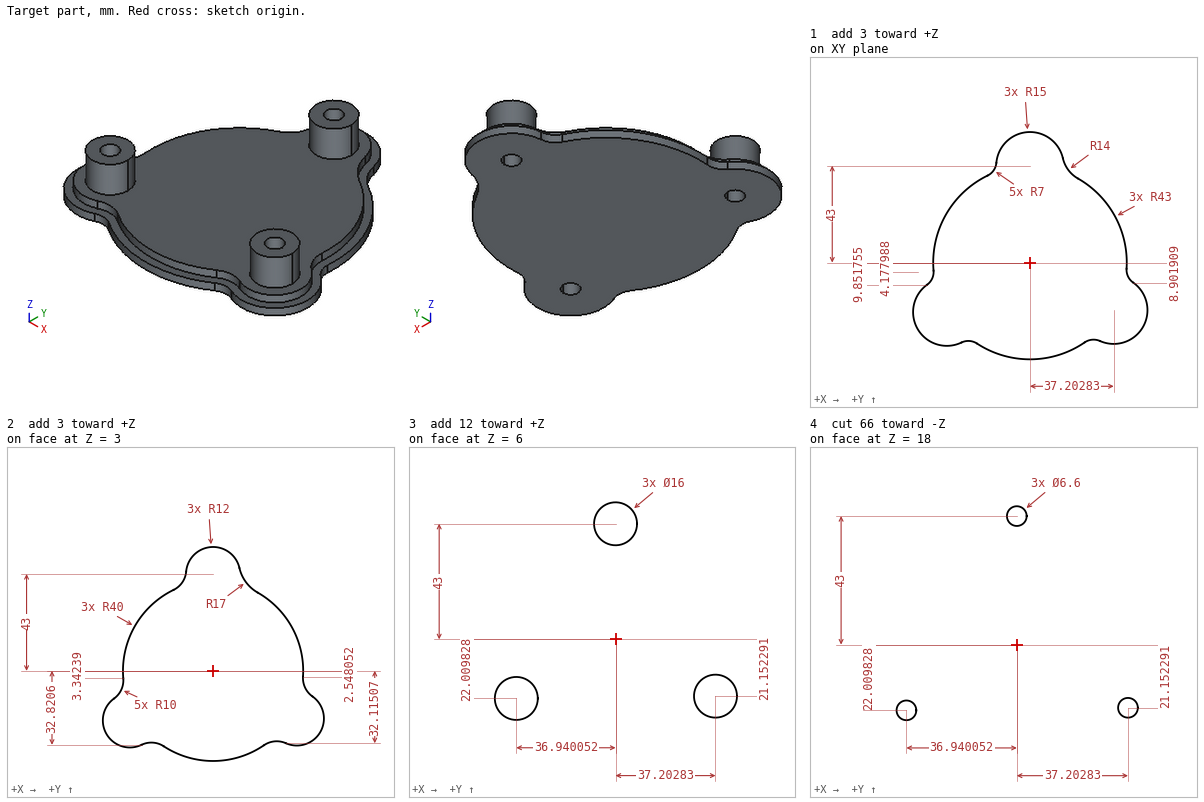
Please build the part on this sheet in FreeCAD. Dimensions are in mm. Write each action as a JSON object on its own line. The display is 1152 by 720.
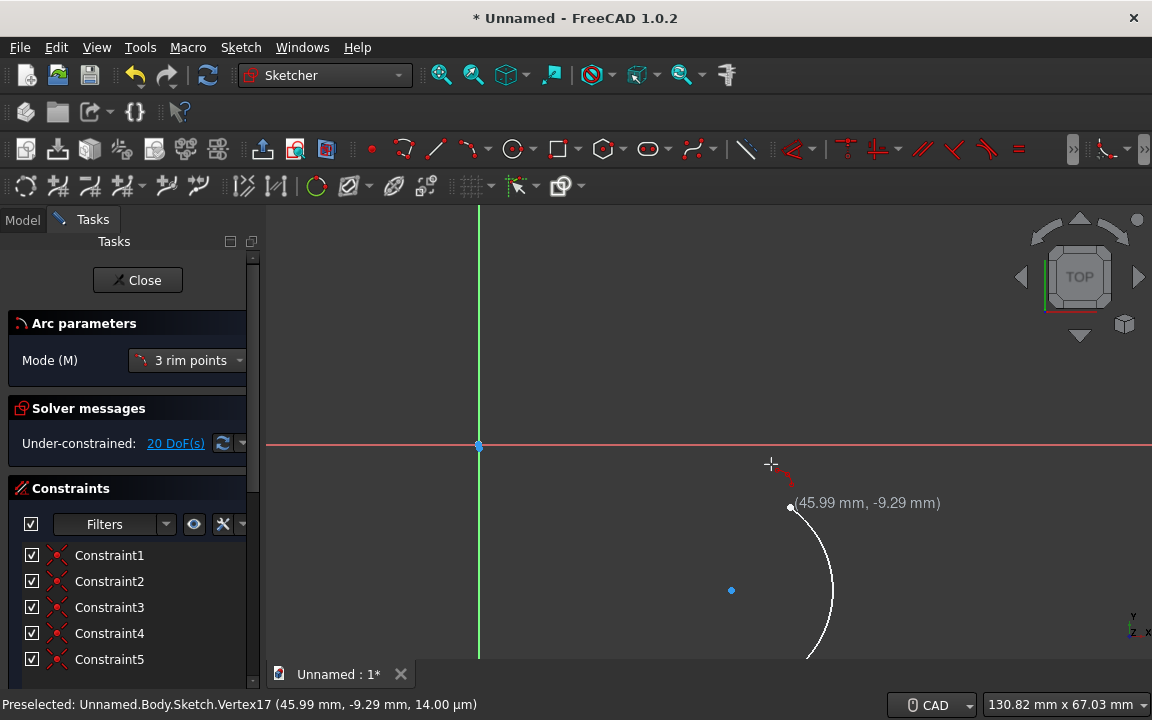
{"action": "left_click", "coordinate": [769, 463]}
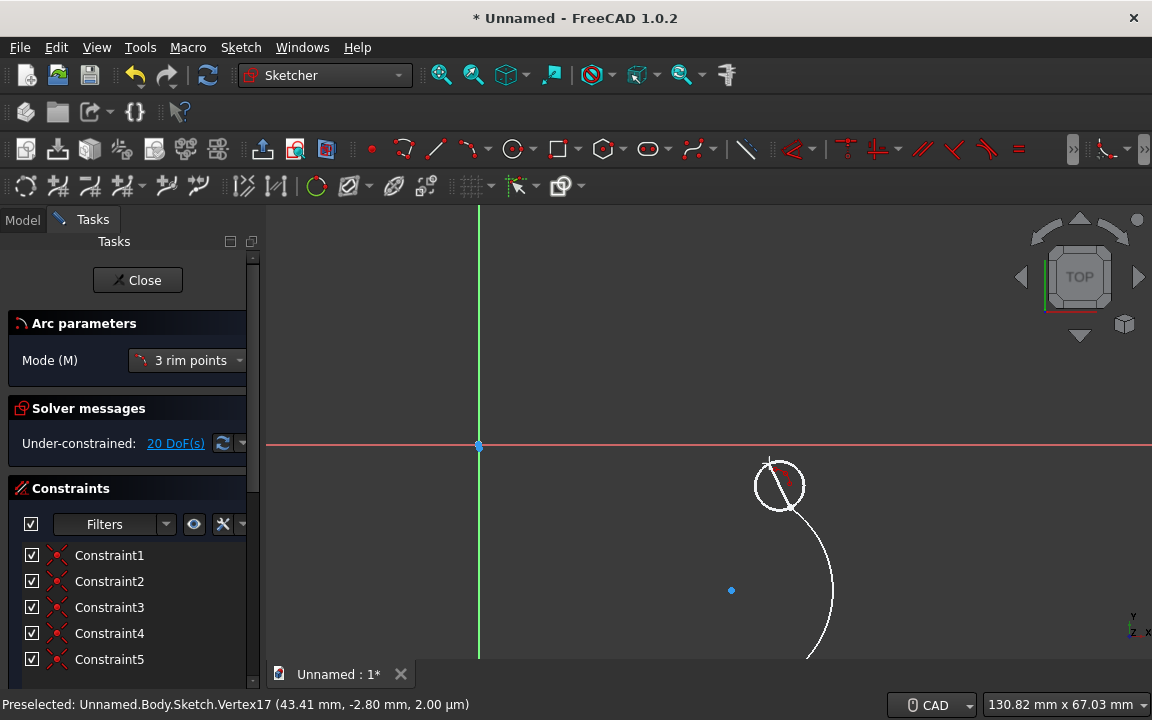
{"action": "scroll", "coordinate": [774, 487], "scroll_direction": "up", "scroll_amount": 5}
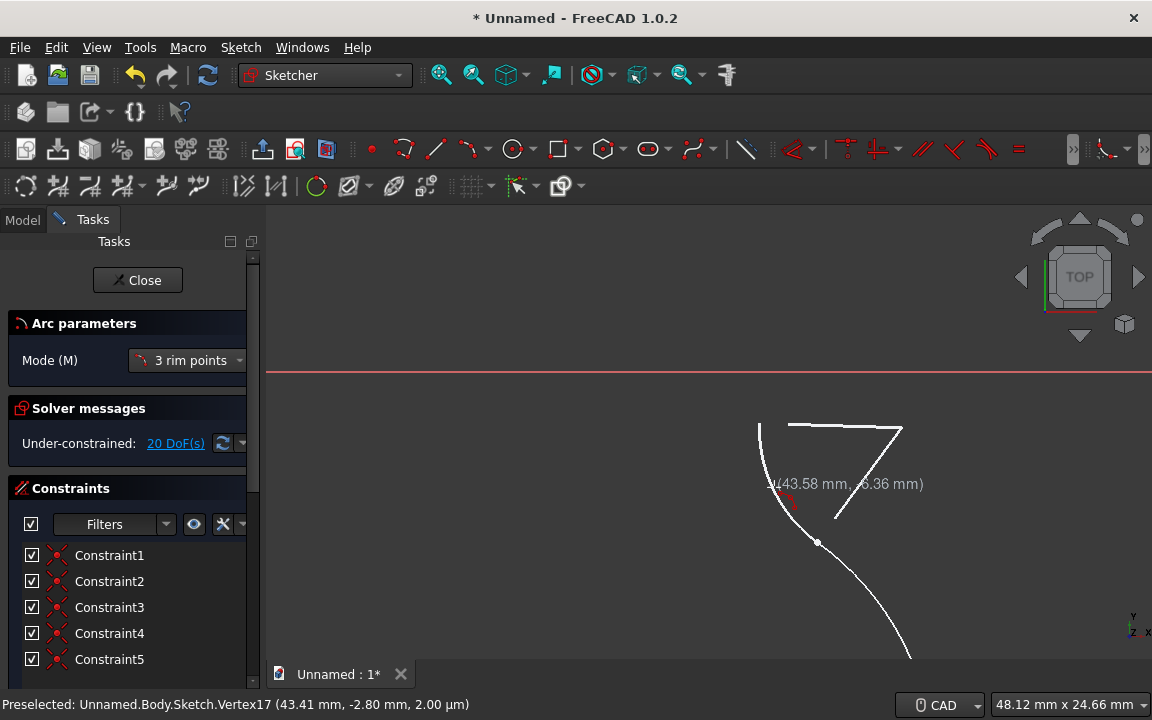
{"action": "left_click", "coordinate": [773, 486]}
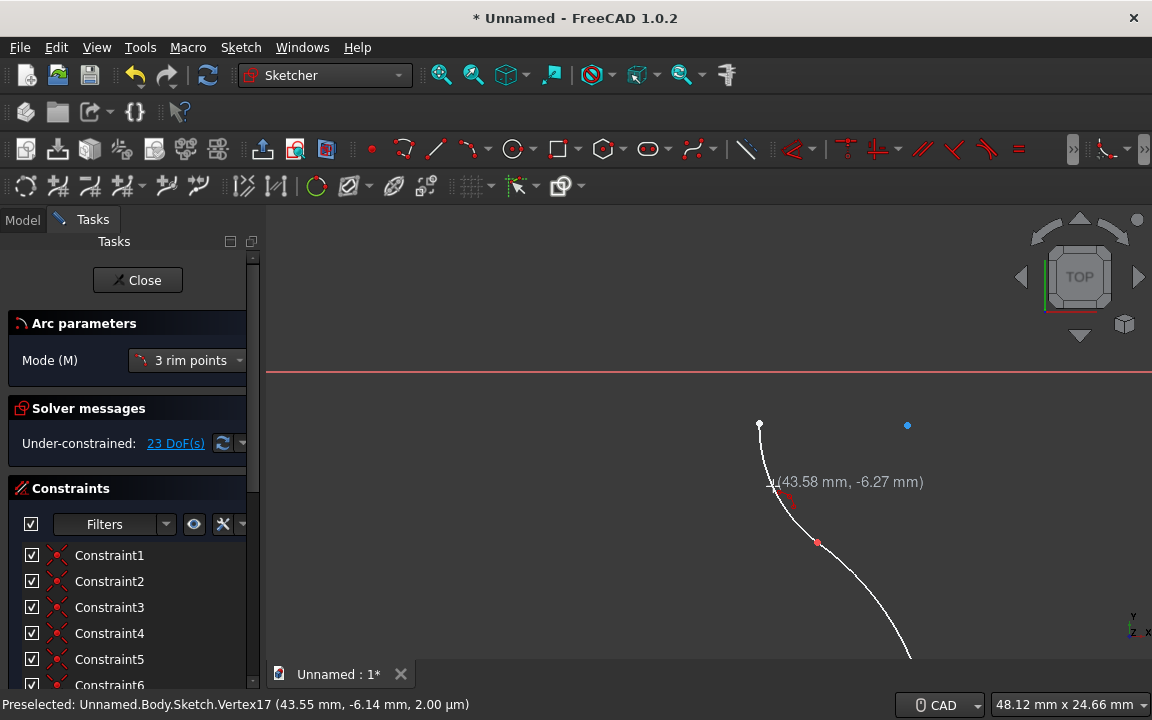
{"action": "scroll", "coordinate": [772, 471], "scroll_direction": "down", "scroll_amount": 9}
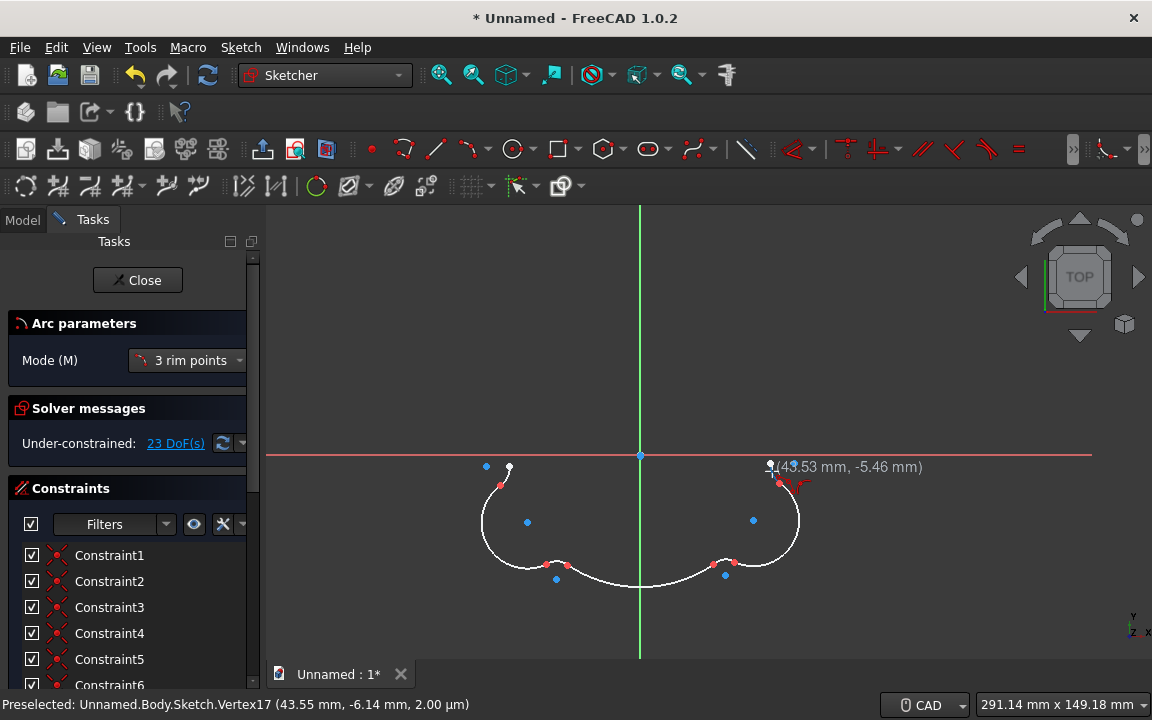
{"action": "scroll", "coordinate": [771, 463], "scroll_direction": "up", "scroll_amount": 4}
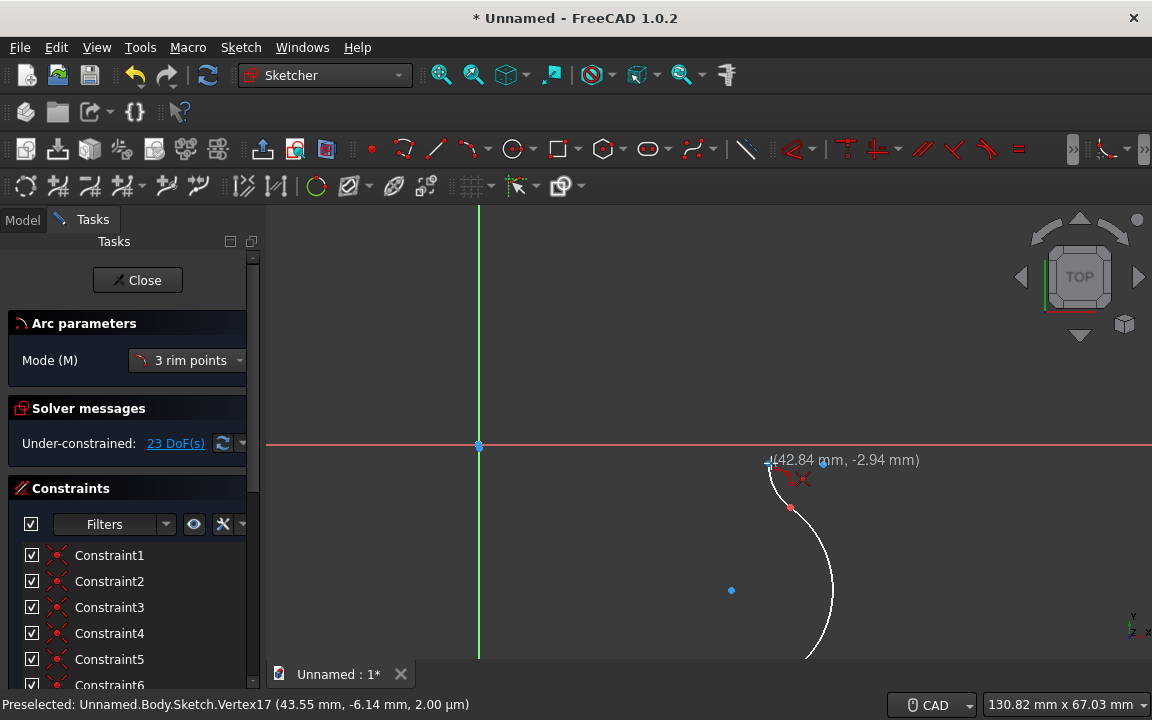
{"action": "left_click", "coordinate": [769, 464]}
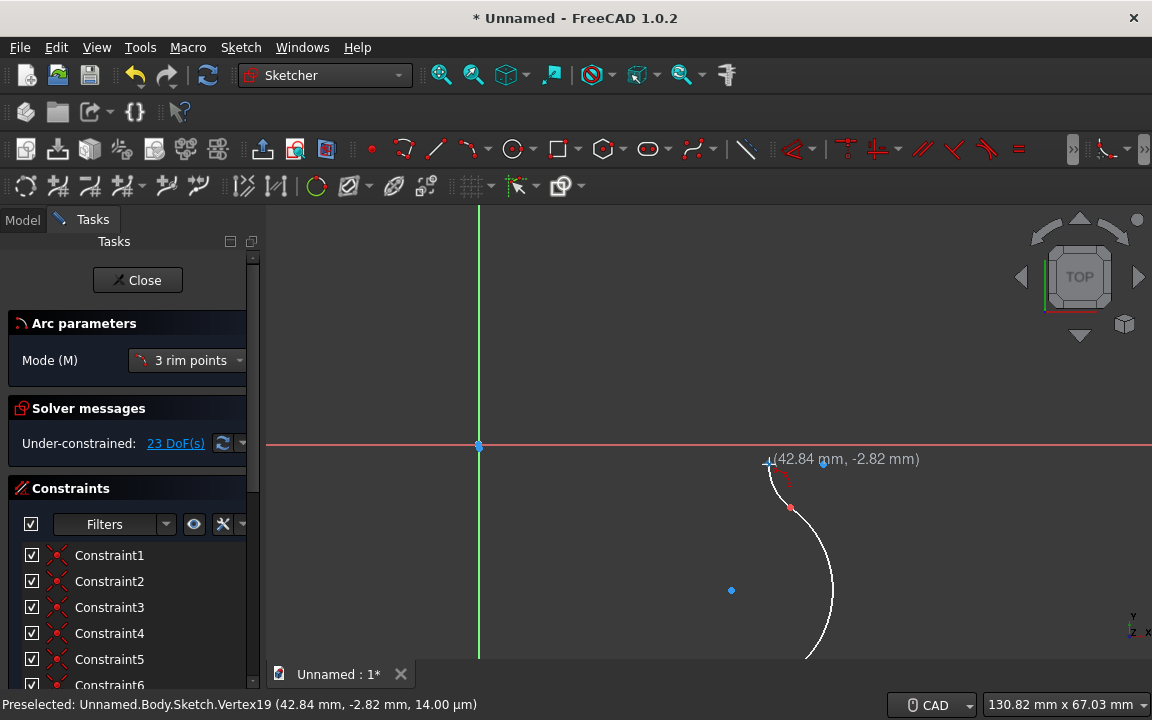
{"action": "scroll", "coordinate": [771, 463], "scroll_direction": "down", "scroll_amount": 4}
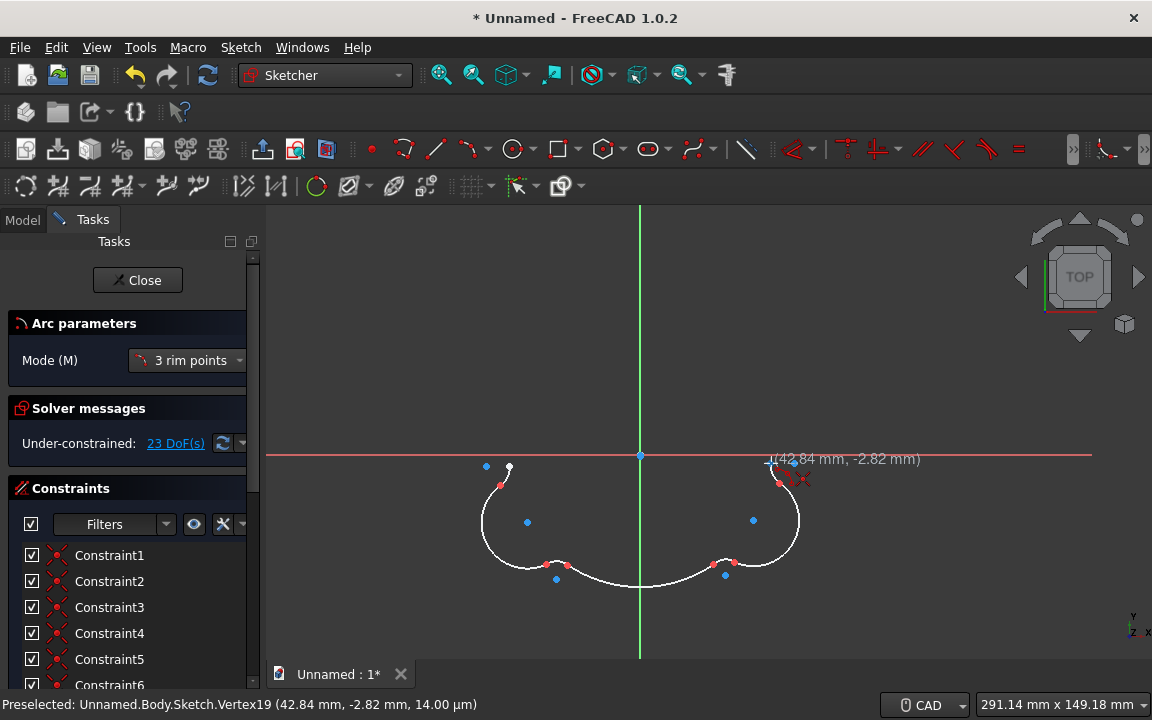
{"action": "left_click", "coordinate": [705, 341]}
{"action": "left_click", "coordinate": [755, 393]}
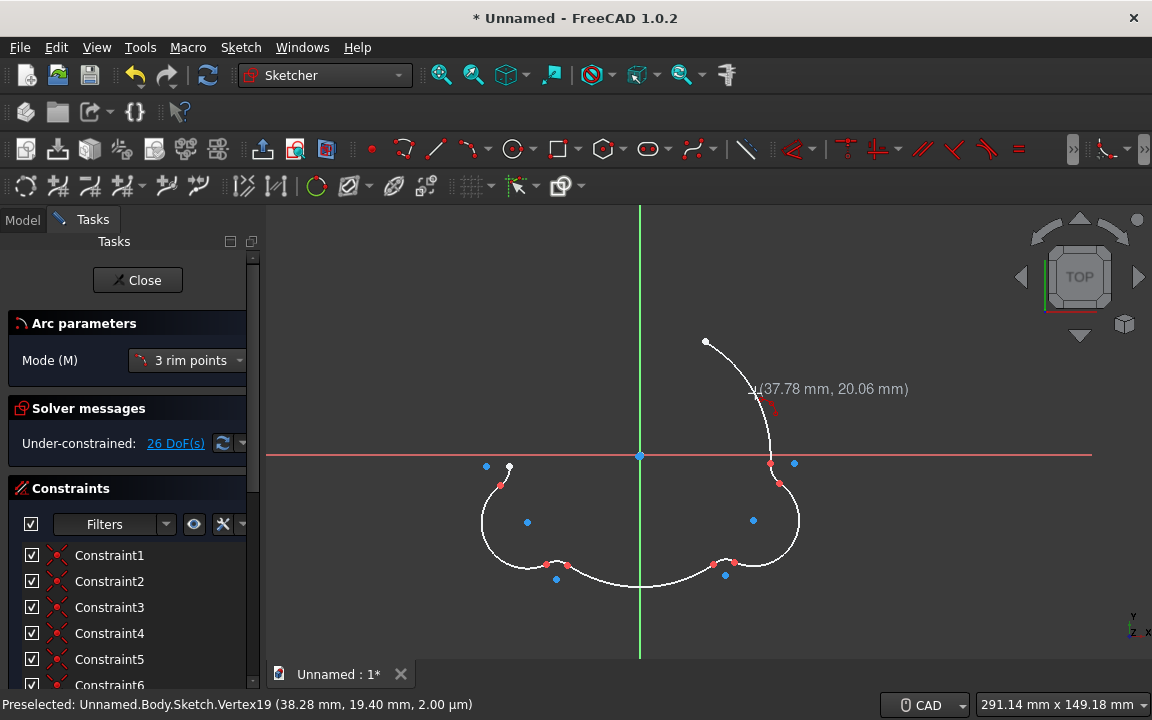
{"action": "left_click", "coordinate": [705, 342]}
{"action": "left_click", "coordinate": [684, 314]}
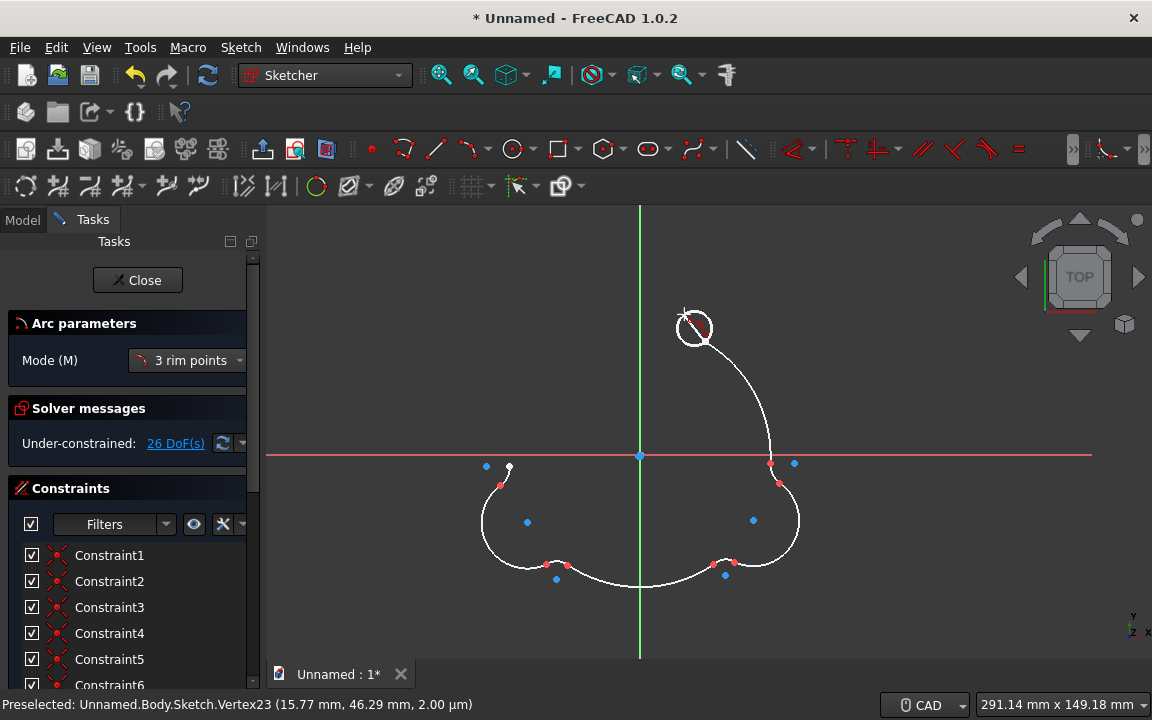
{"action": "scroll", "coordinate": [692, 330], "scroll_direction": "up", "scroll_amount": 8}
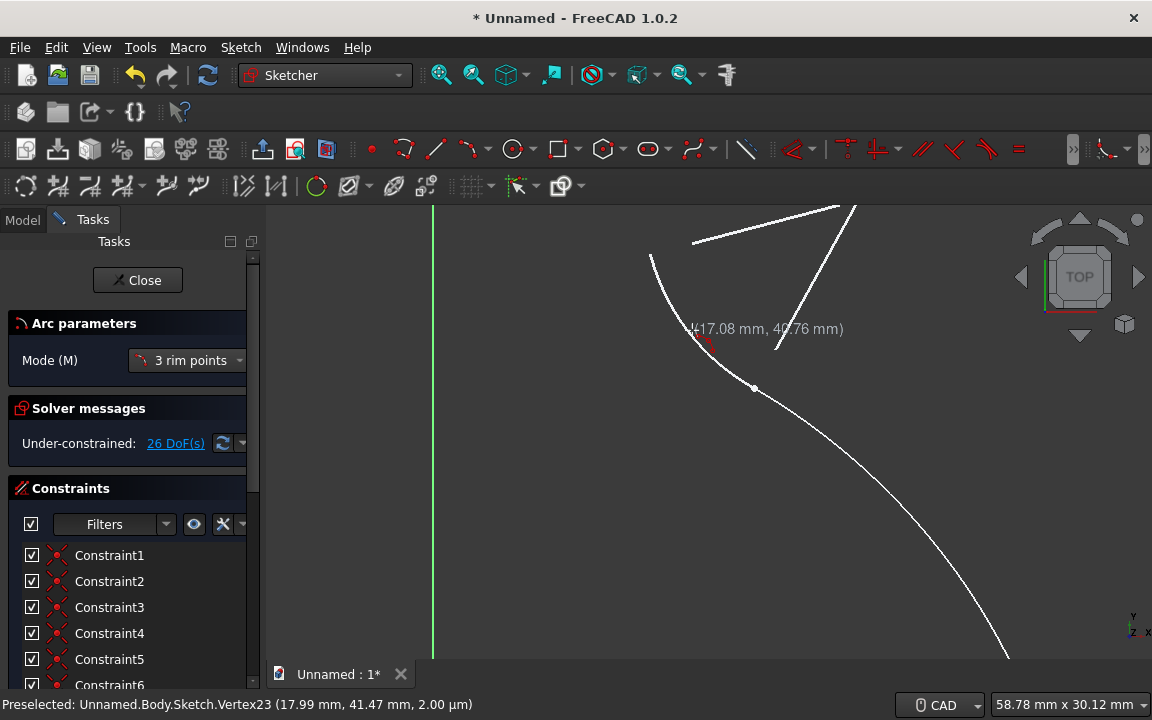
{"action": "left_click", "coordinate": [689, 328]}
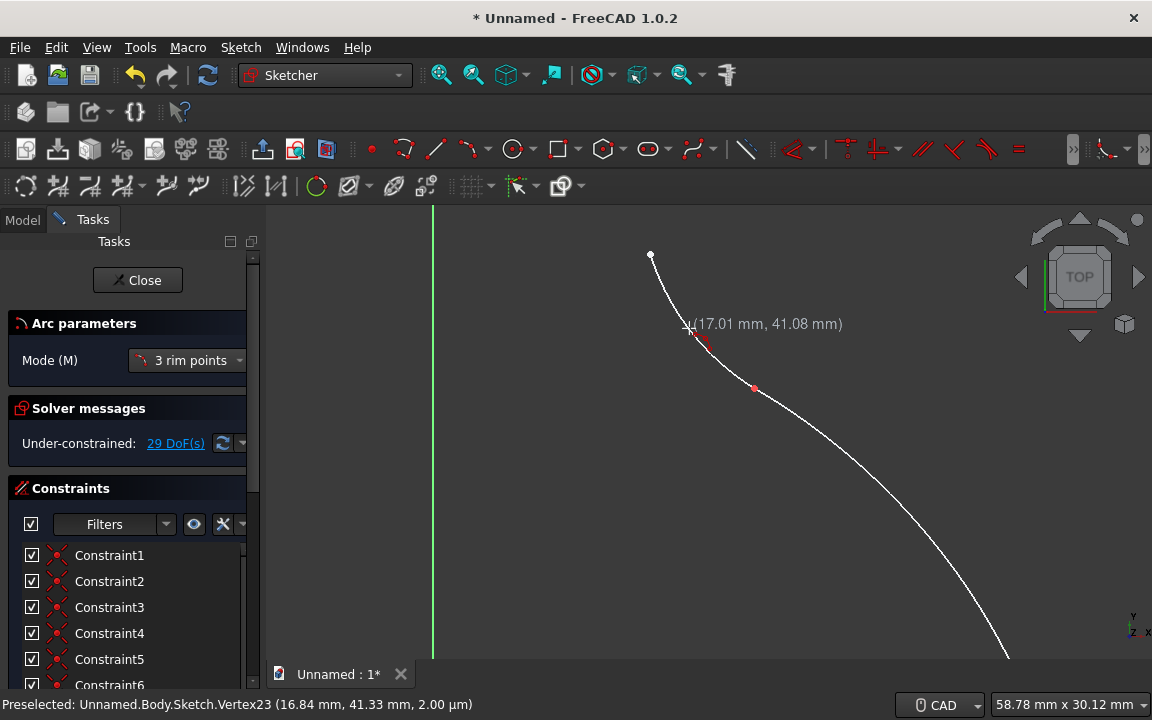
{"action": "scroll", "coordinate": [692, 330], "scroll_direction": "down", "scroll_amount": 8}